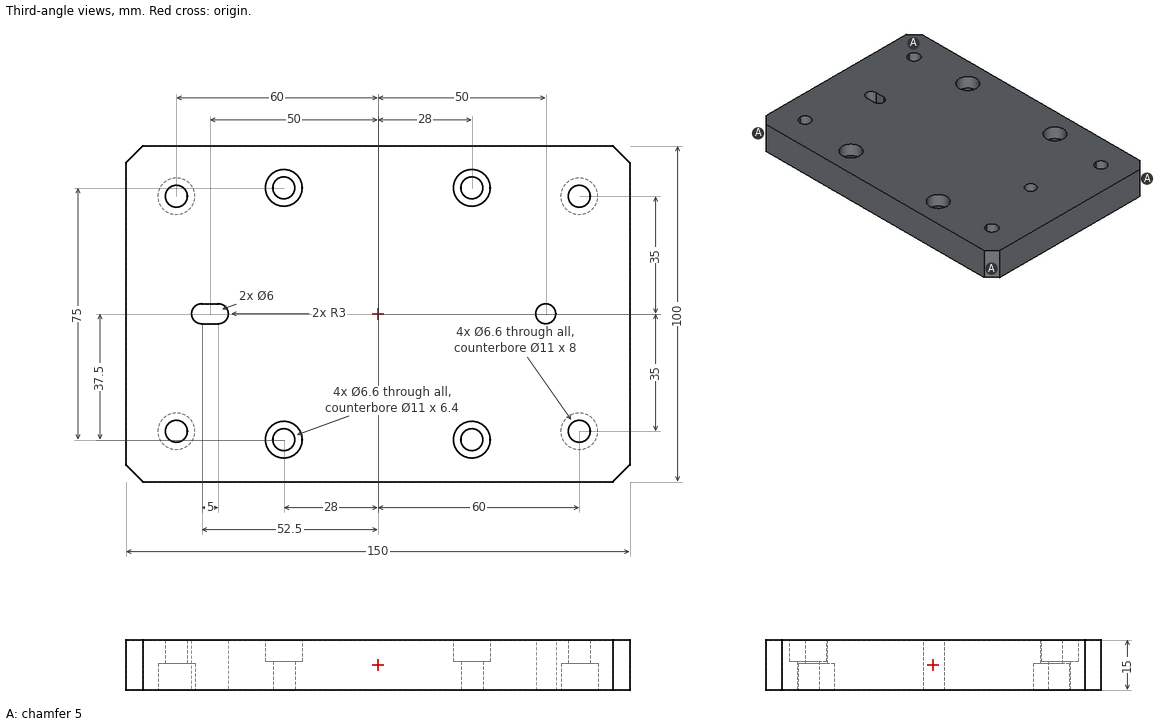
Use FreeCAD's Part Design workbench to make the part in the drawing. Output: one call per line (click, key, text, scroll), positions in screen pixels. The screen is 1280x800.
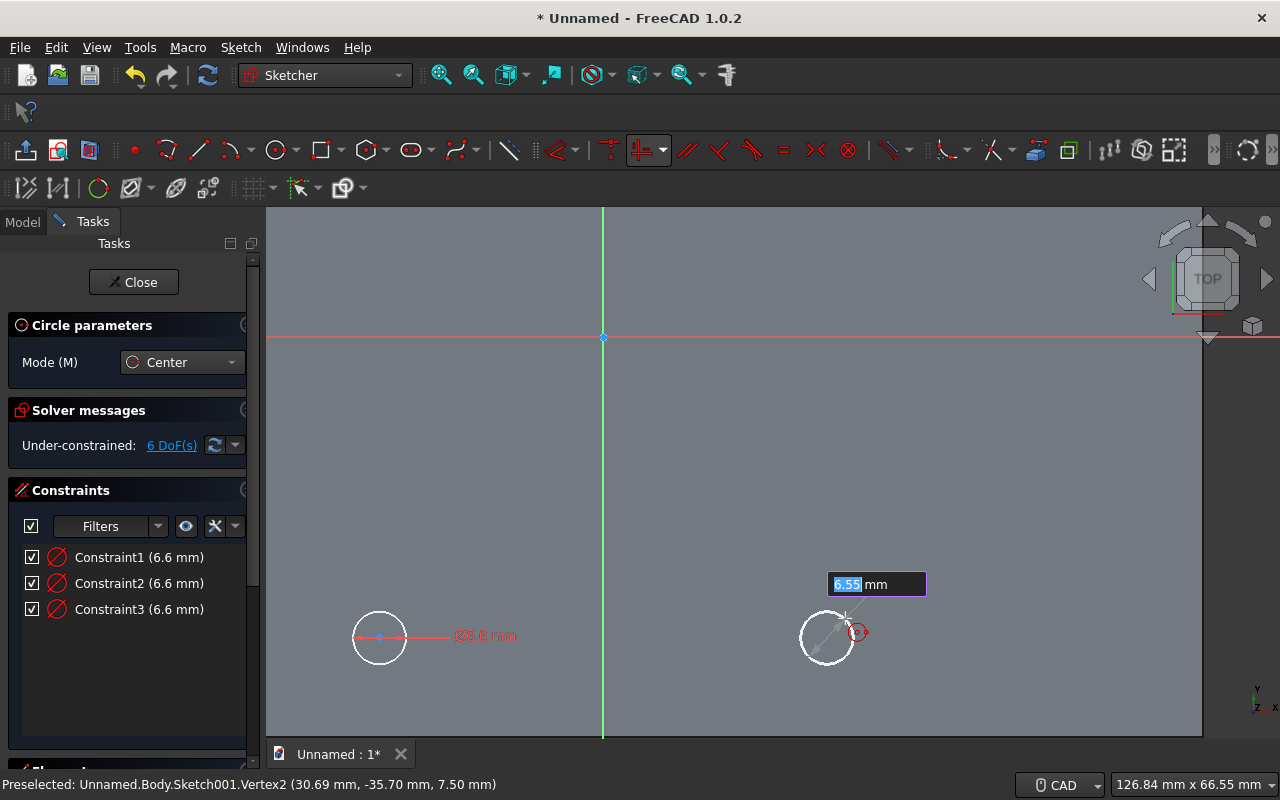
text(6.6)
key(Return)
key(Escape)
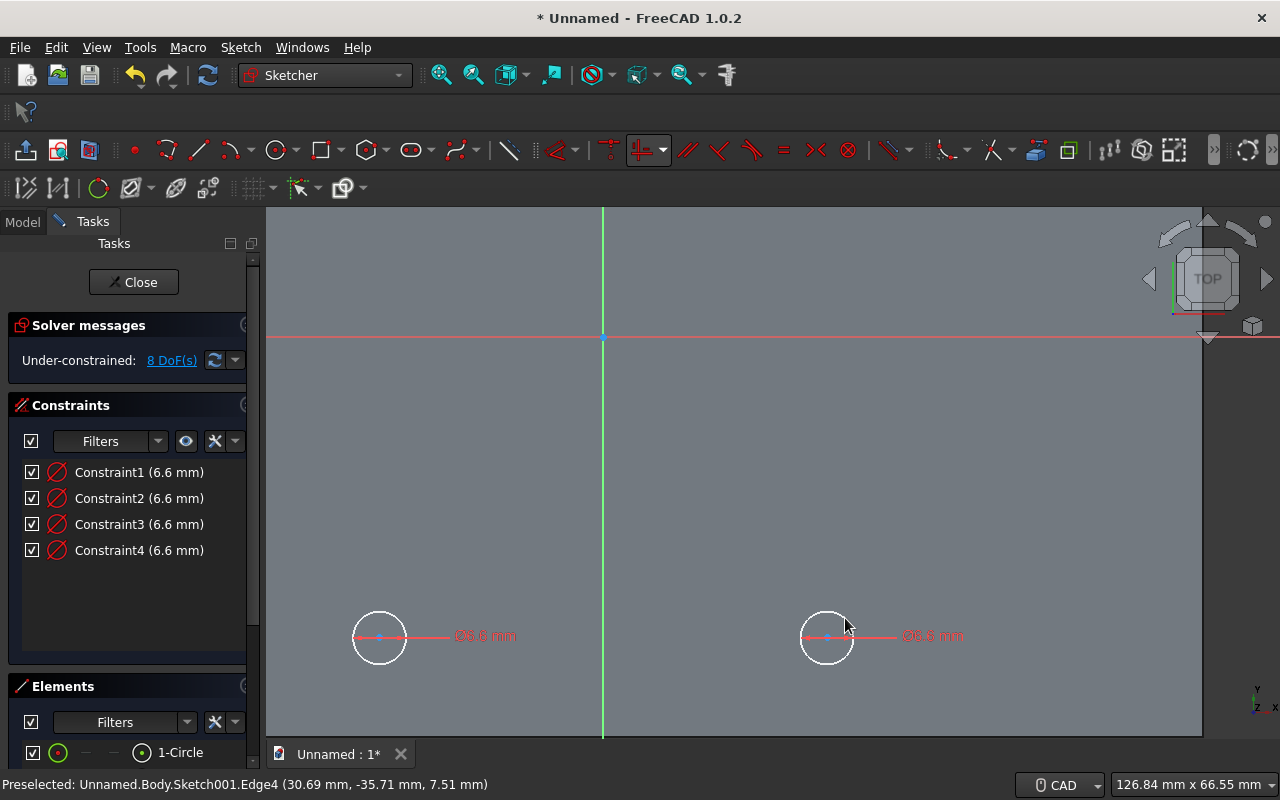
click(380, 638)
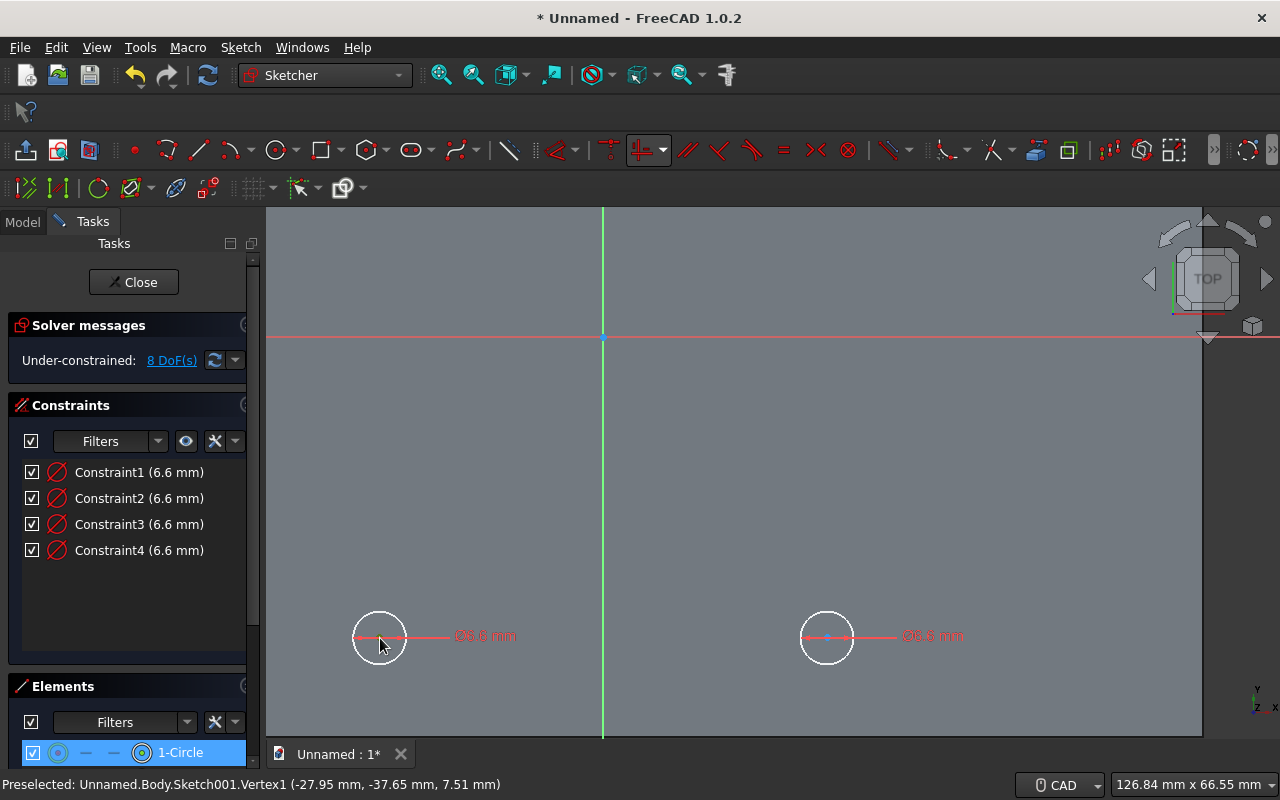
scroll(828, 638, down, 3)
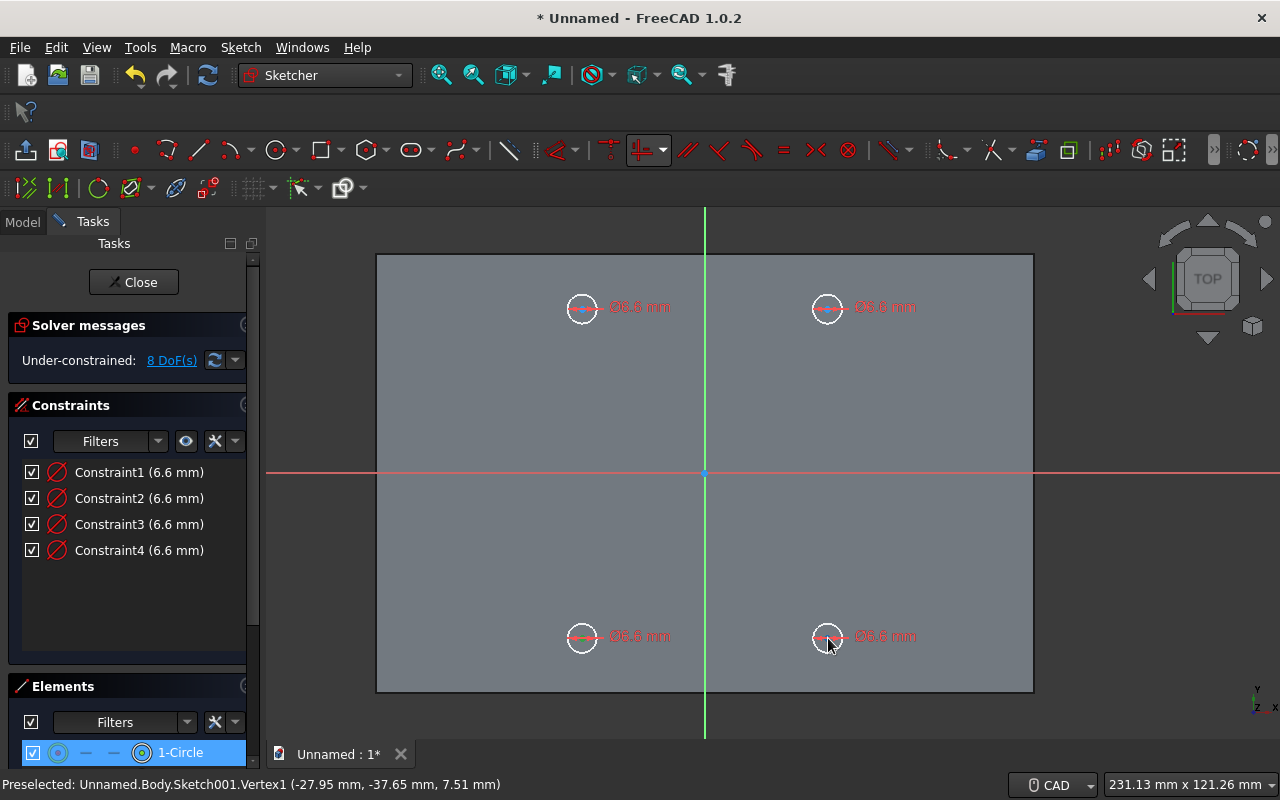
click(582, 309)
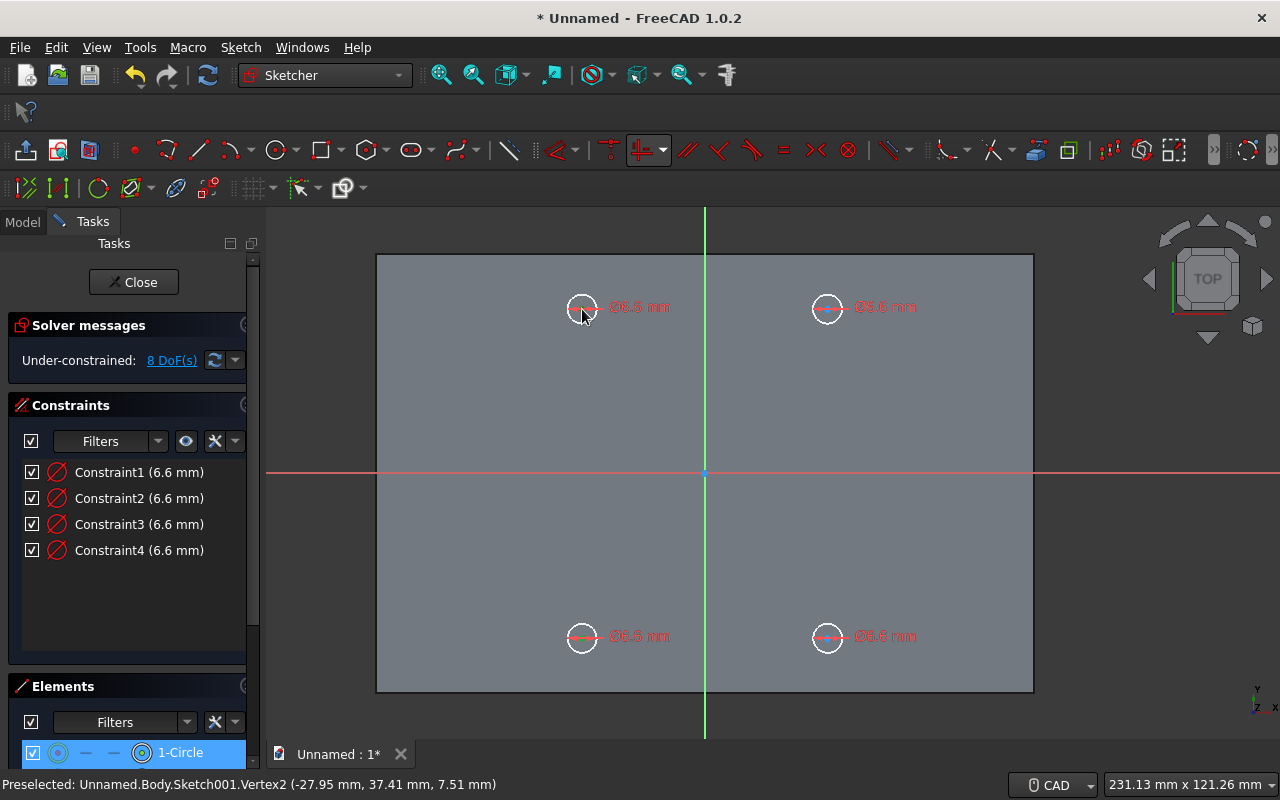
key(v)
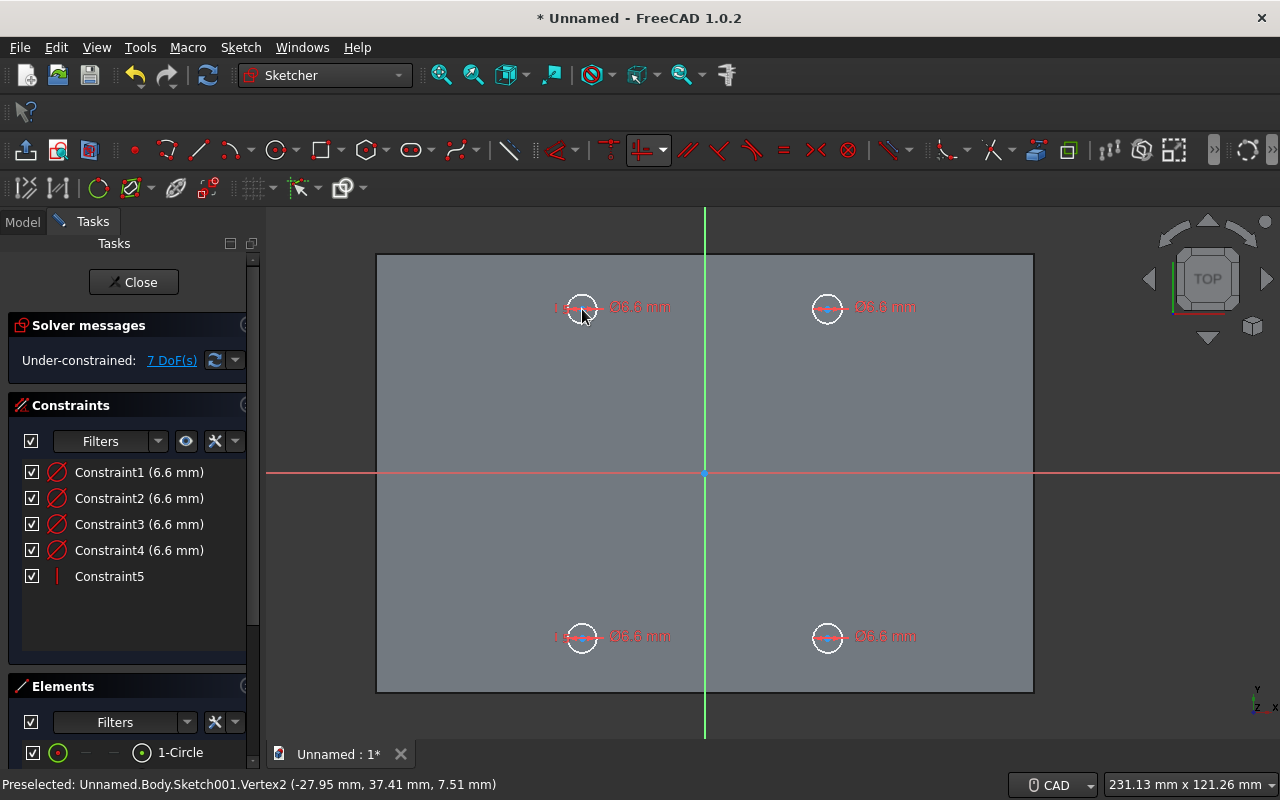
click(582, 309)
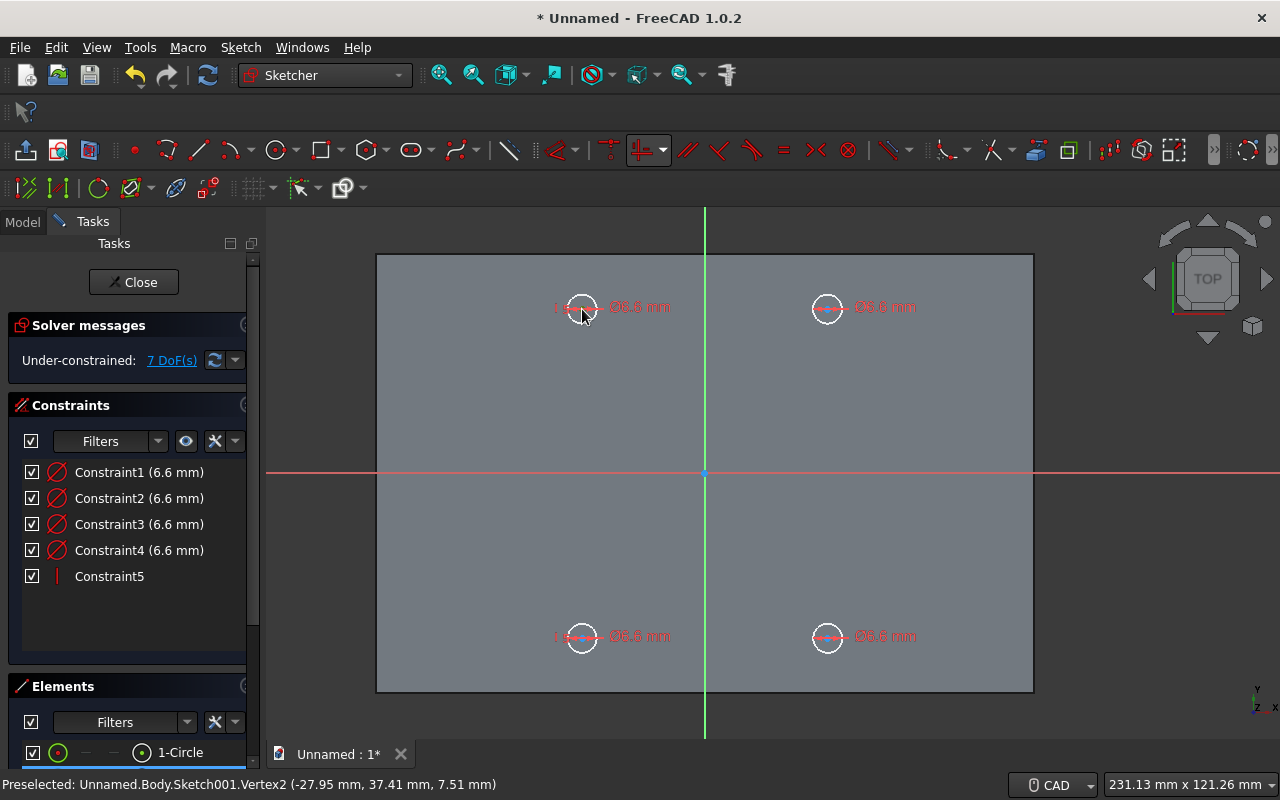
click(827, 309)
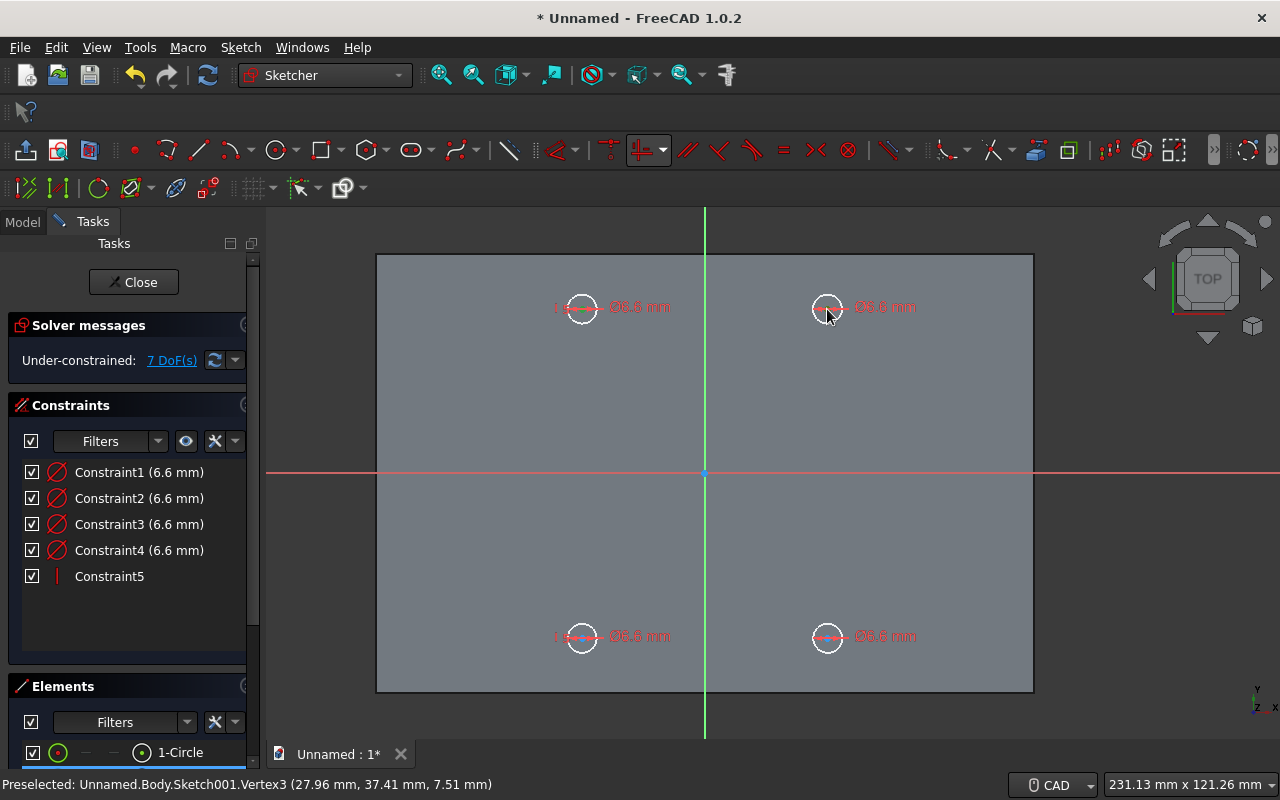
key(h)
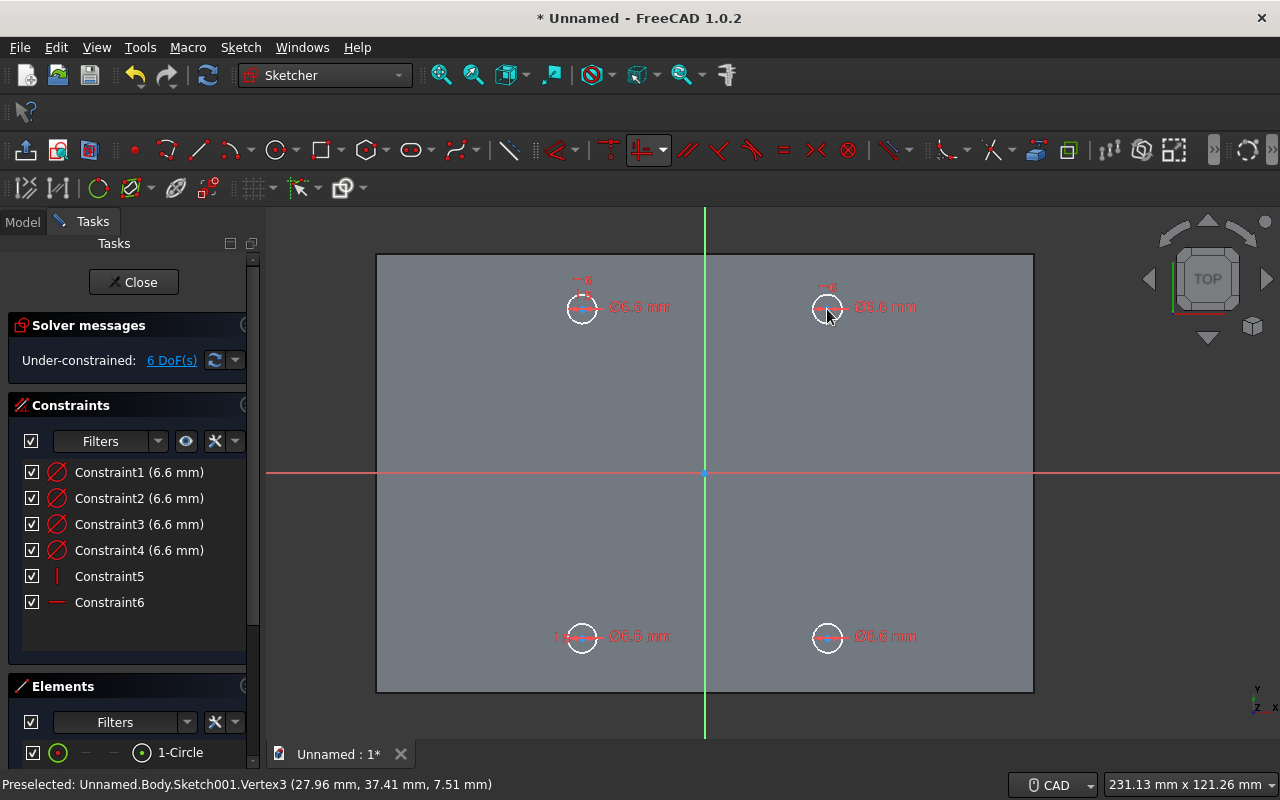
click(827, 309)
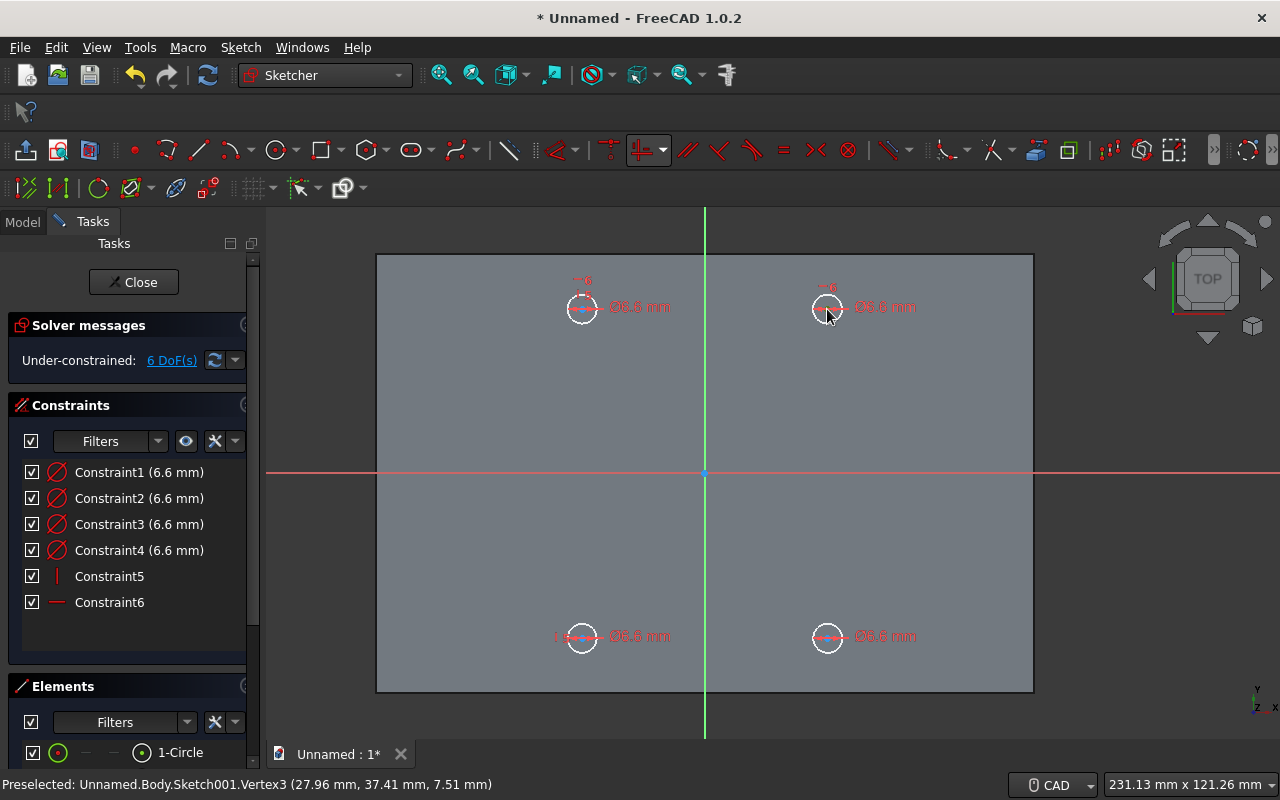
click(828, 638)